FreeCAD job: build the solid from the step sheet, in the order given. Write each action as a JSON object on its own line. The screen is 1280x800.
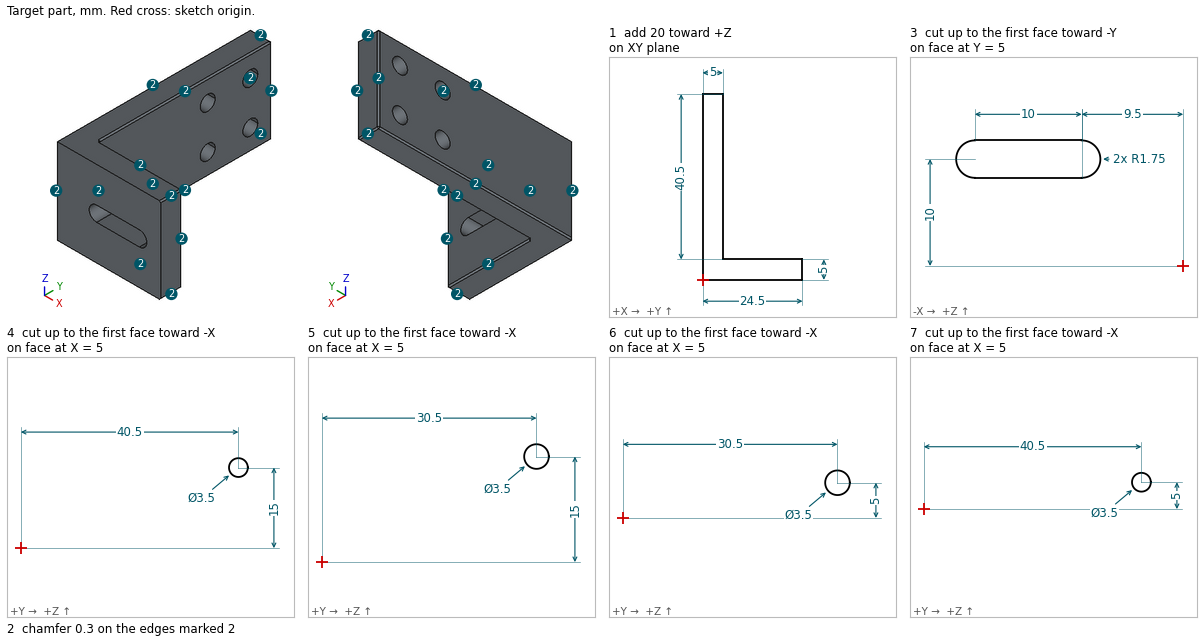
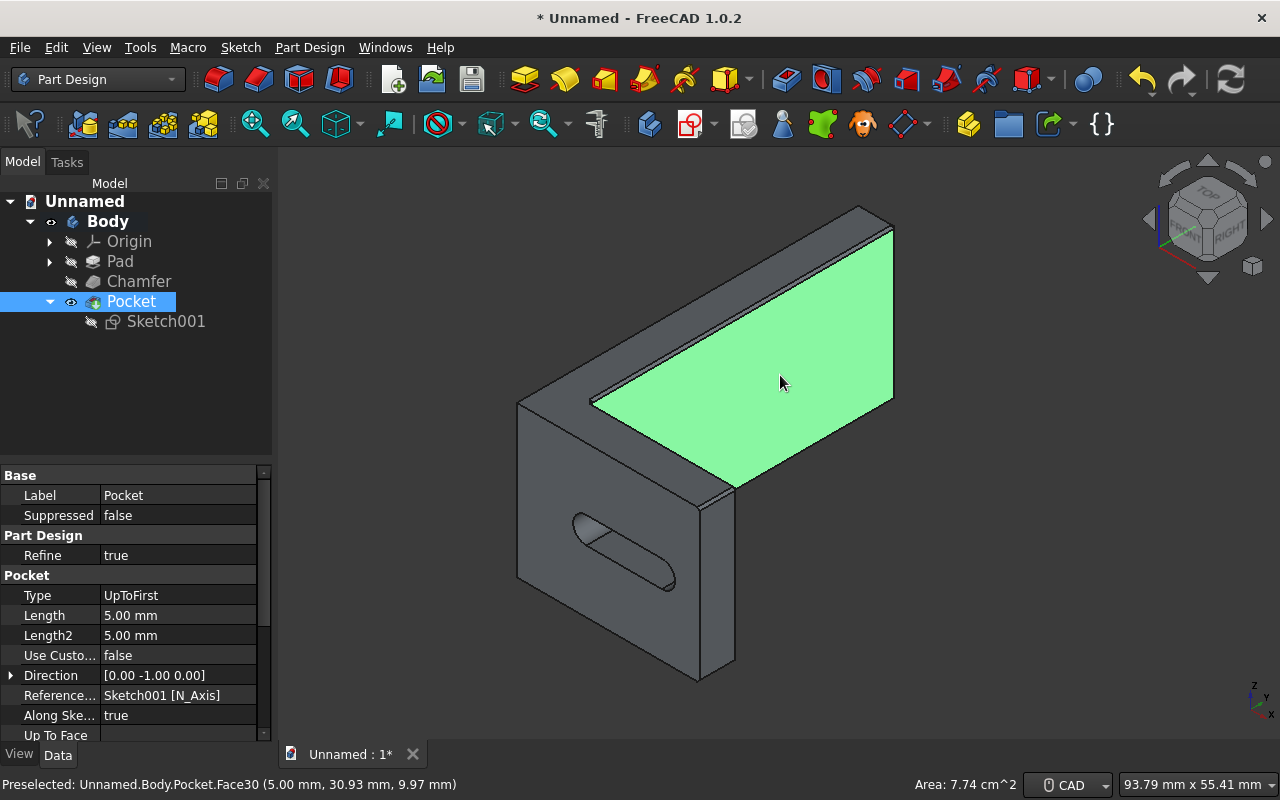
{"action": "left_click", "coordinate": [690, 124]}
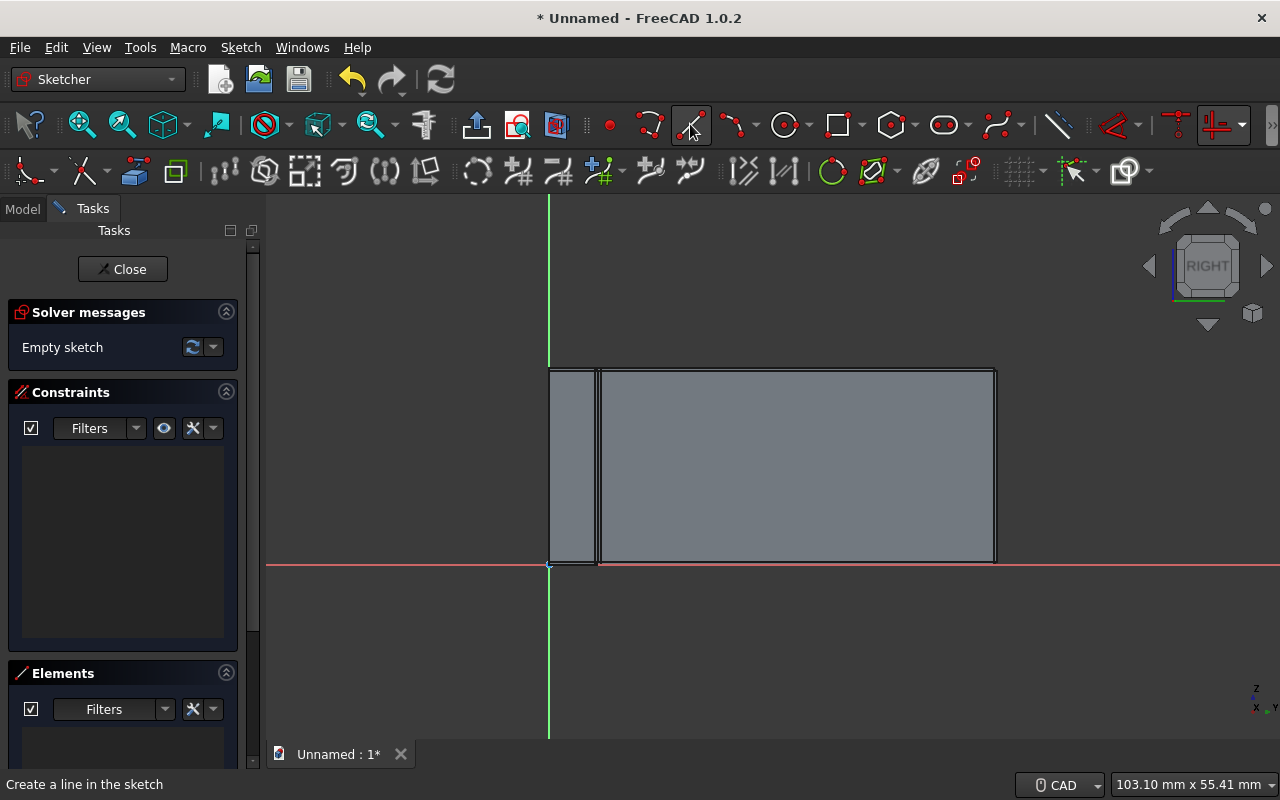
{"action": "key", "text": "q s"}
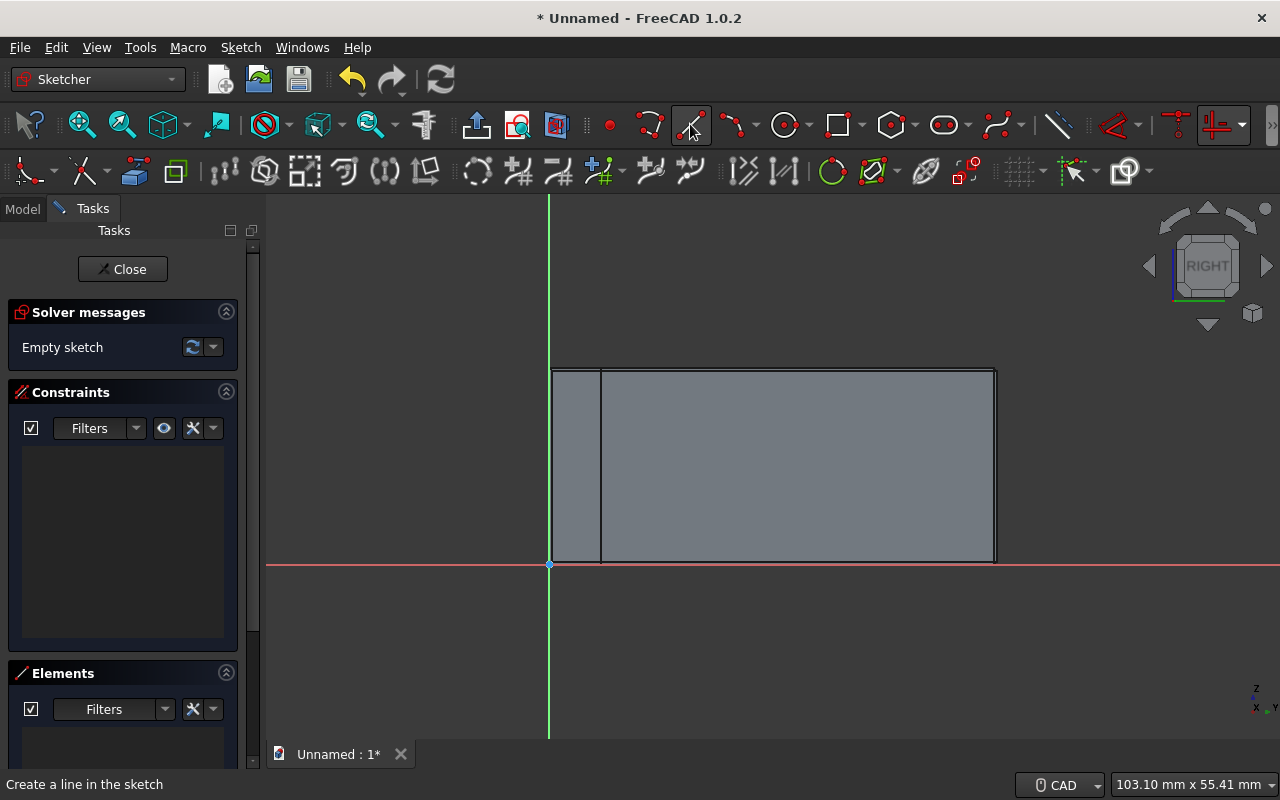
{"action": "scroll", "coordinate": [972, 412], "scroll_direction": "up", "scroll_amount": 12}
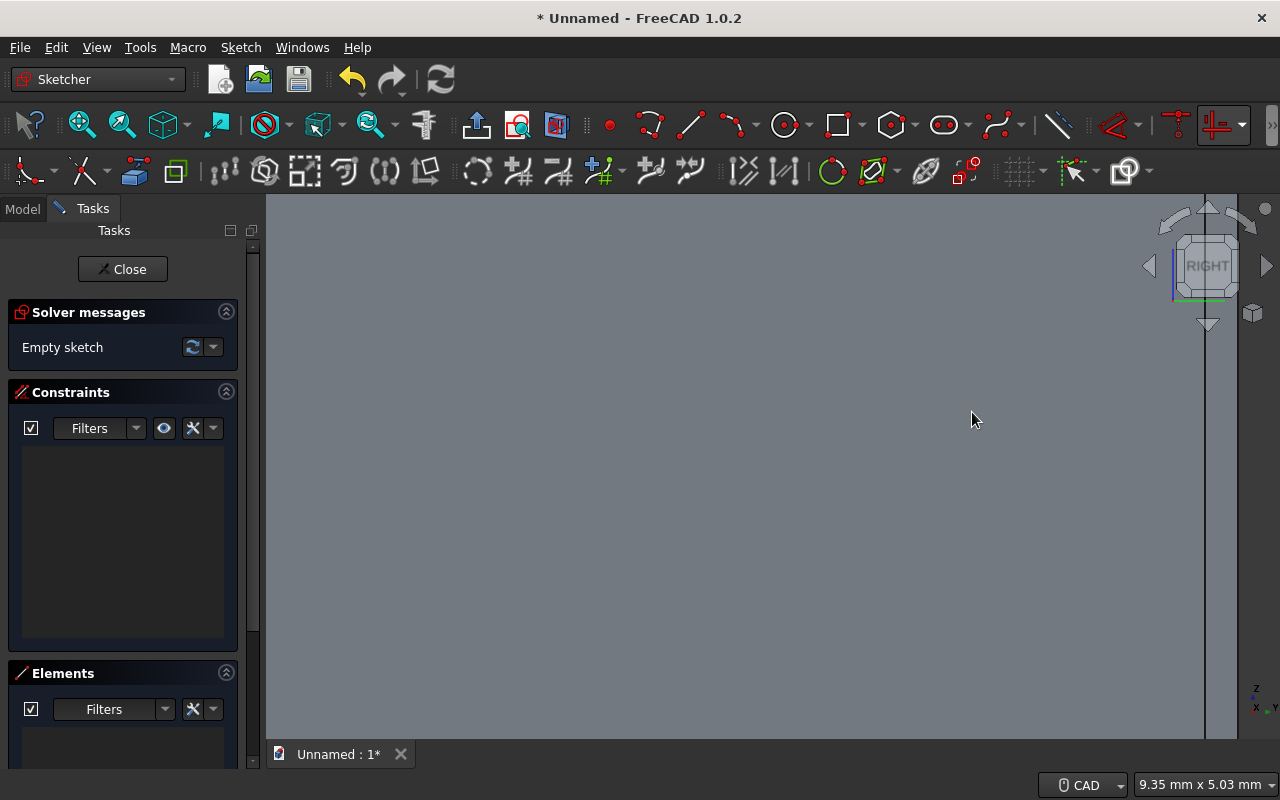
{"action": "left_click", "coordinate": [786, 126]}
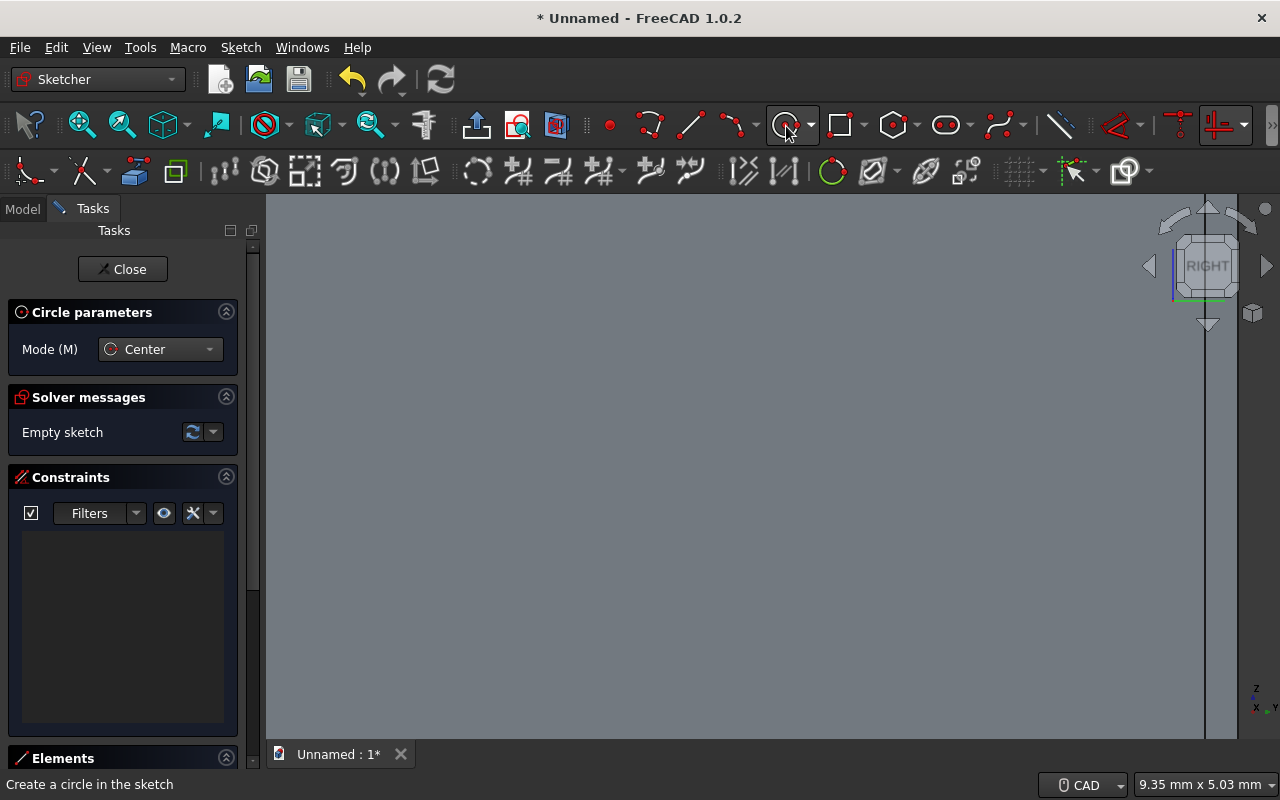
{"action": "left_click", "coordinate": [696, 467]}
{"action": "left_click", "coordinate": [830, 333]}
{"action": "key", "text": "Escape"}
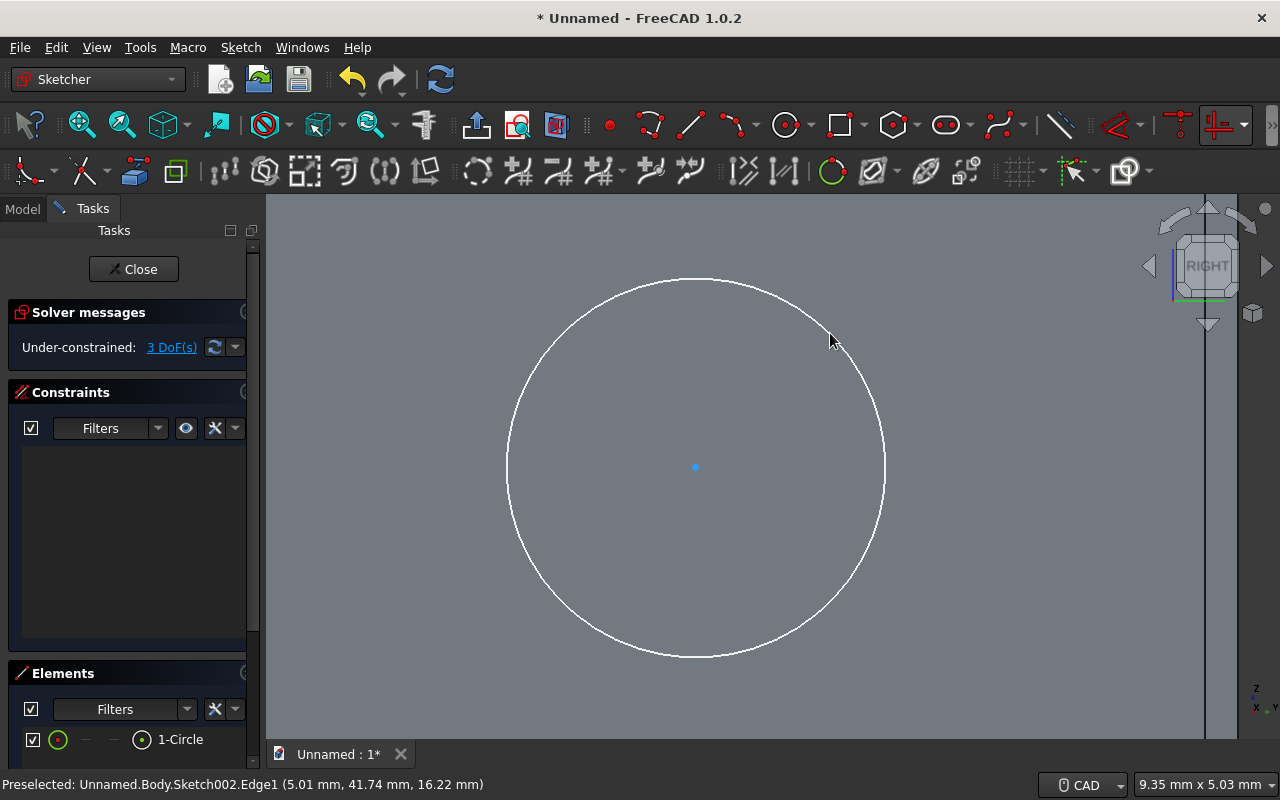
{"action": "left_click", "coordinate": [1116, 126]}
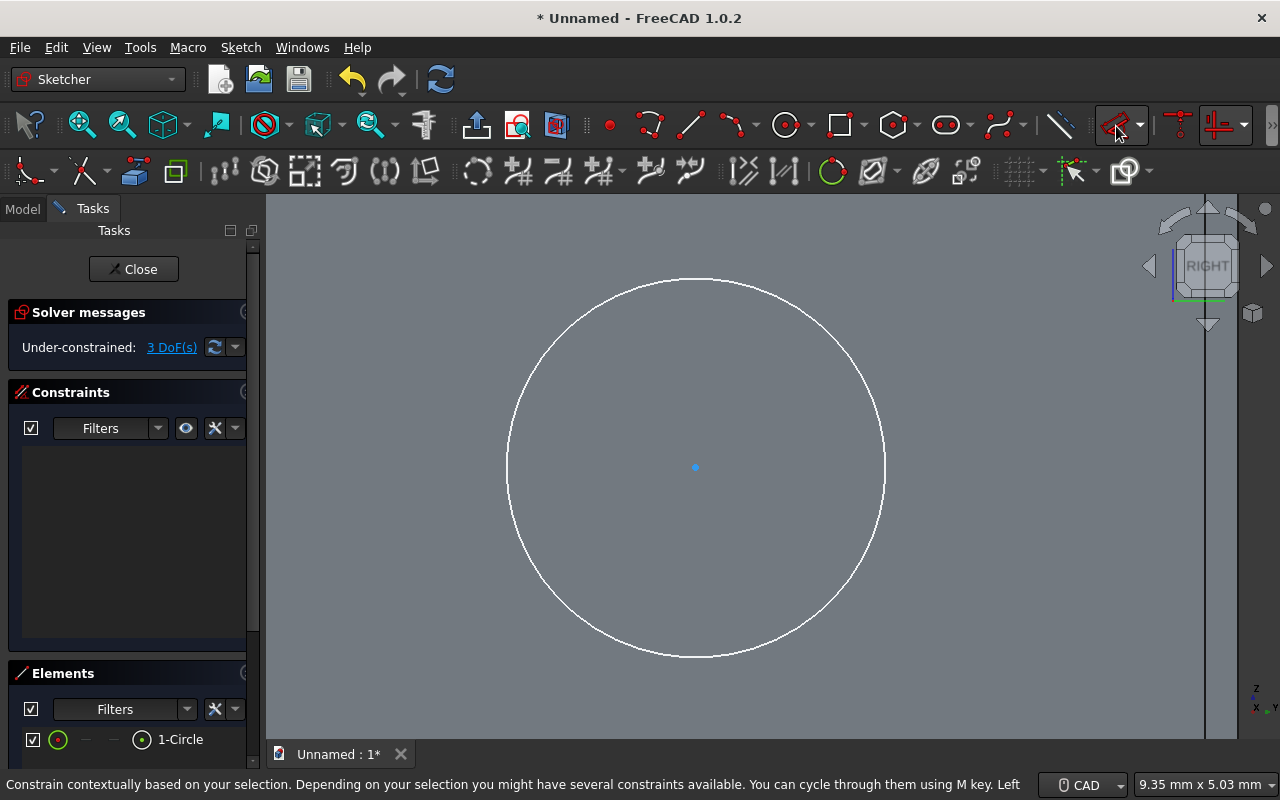
{"action": "left_click", "coordinate": [830, 334]}
{"action": "left_click", "coordinate": [853, 311]}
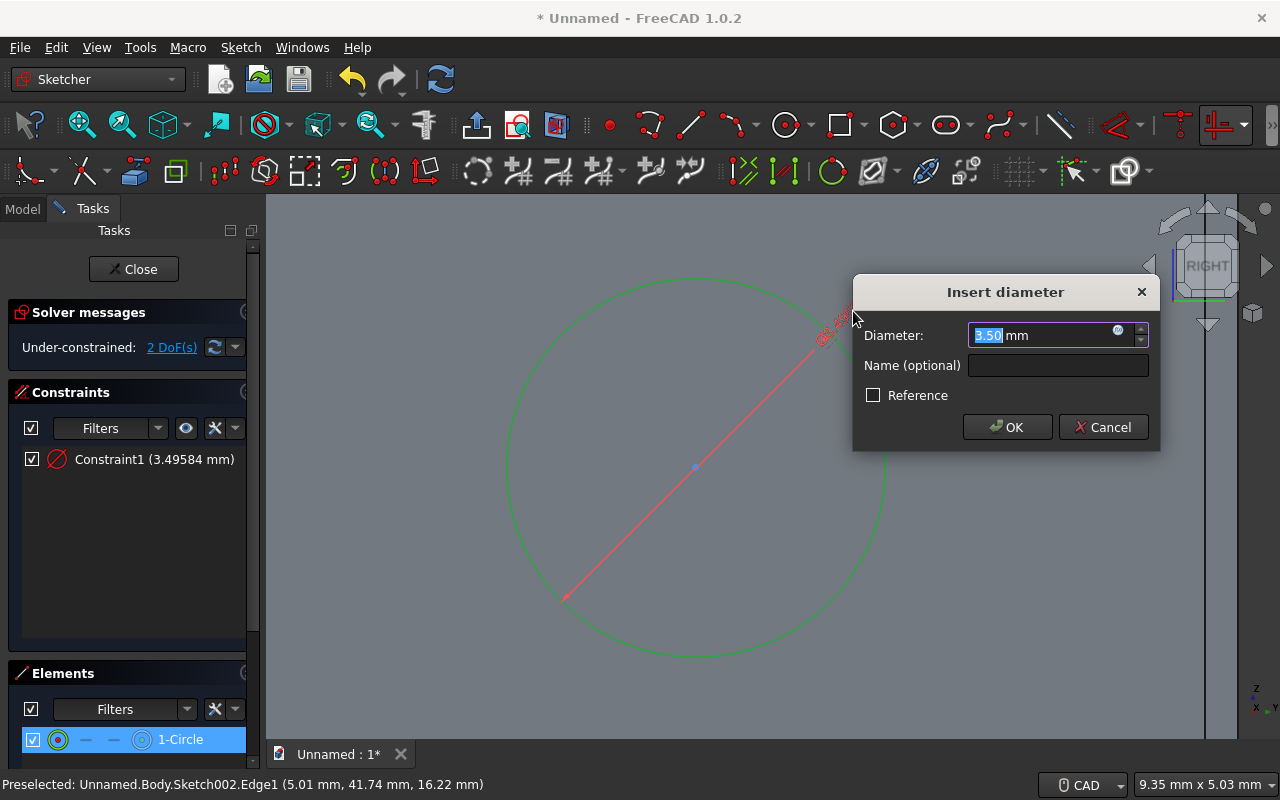
{"action": "type", "text": "3.5"}
{"action": "key", "text": "Return"}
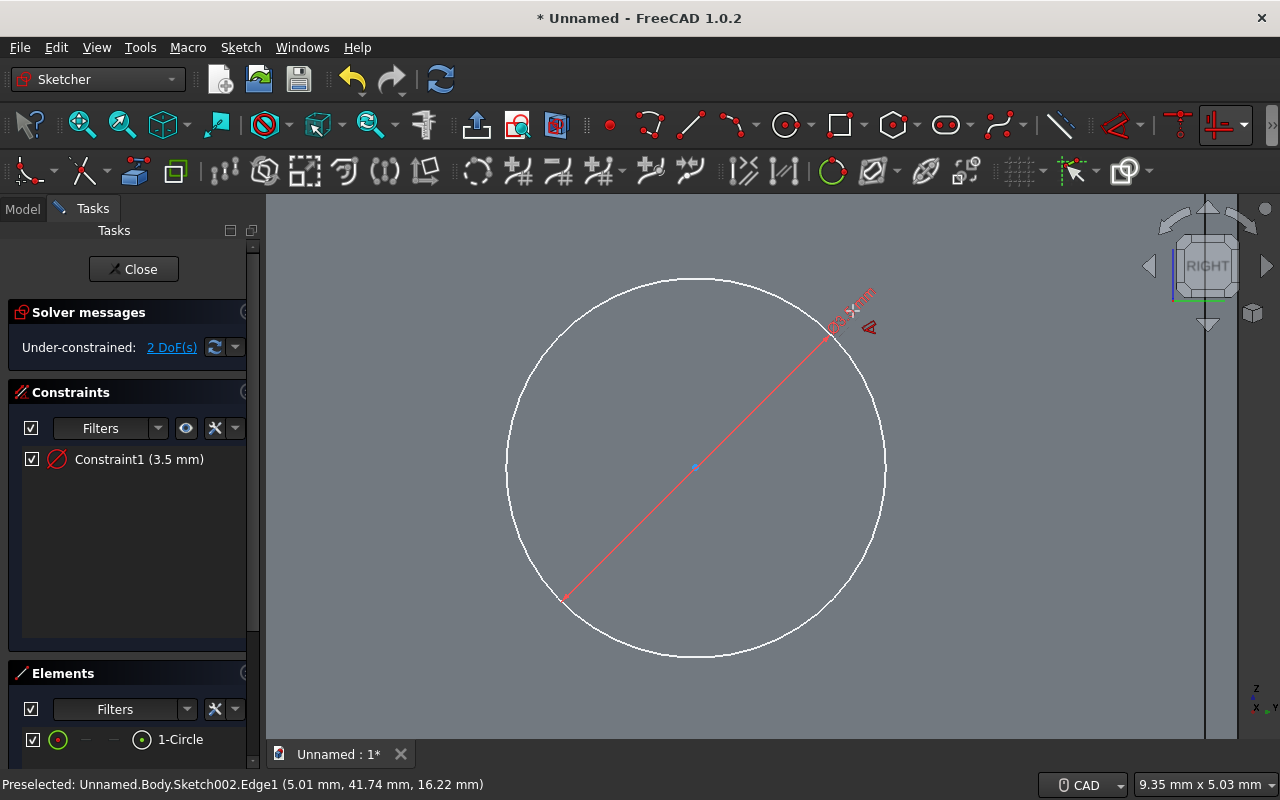
{"action": "left_click", "coordinate": [696, 468]}
{"action": "left_click", "coordinate": [730, 589]}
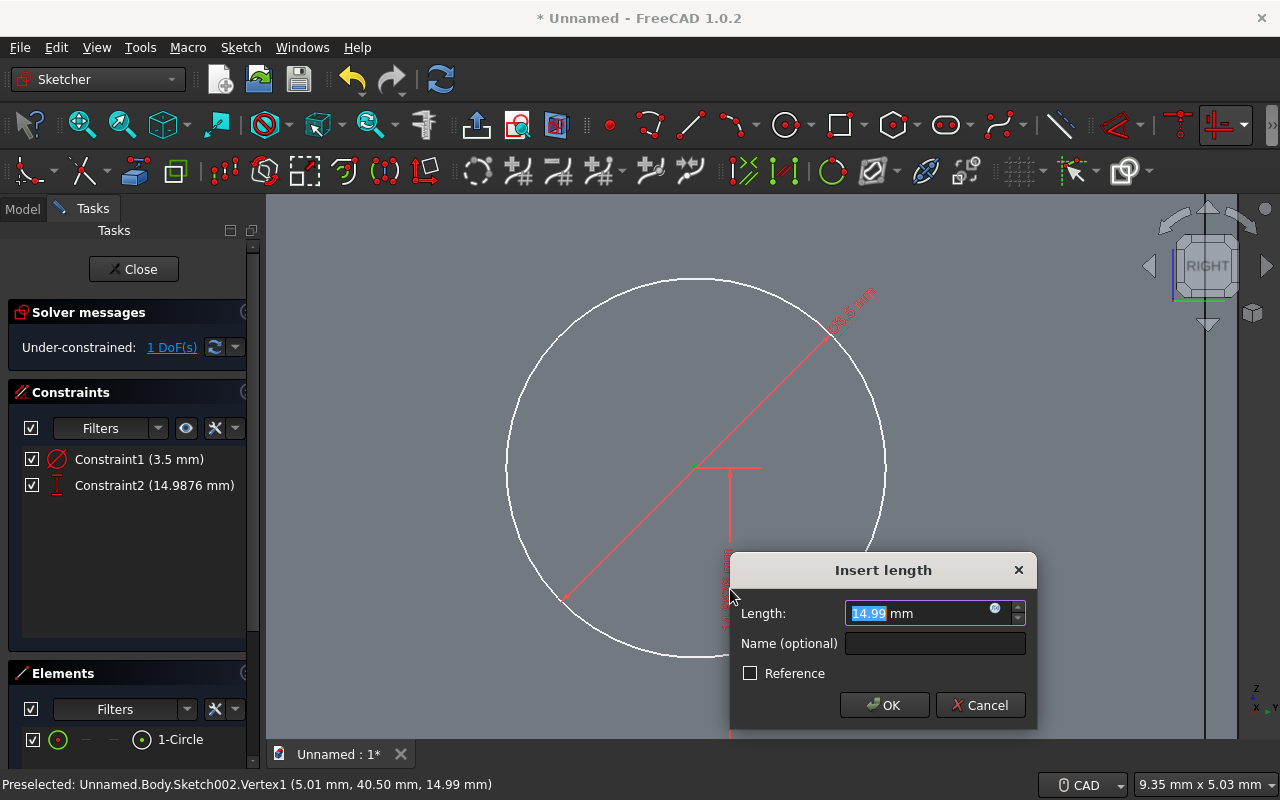
{"action": "type", "text": "15"}
{"action": "key", "text": "Return"}